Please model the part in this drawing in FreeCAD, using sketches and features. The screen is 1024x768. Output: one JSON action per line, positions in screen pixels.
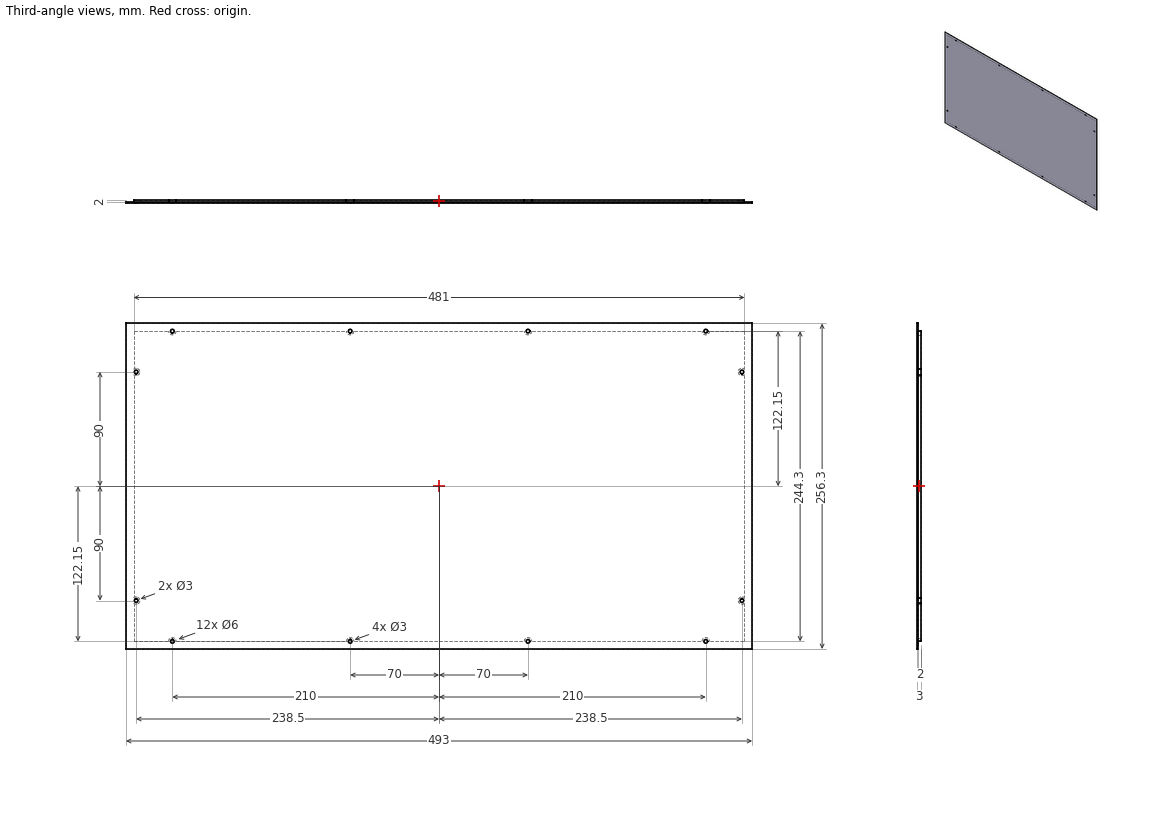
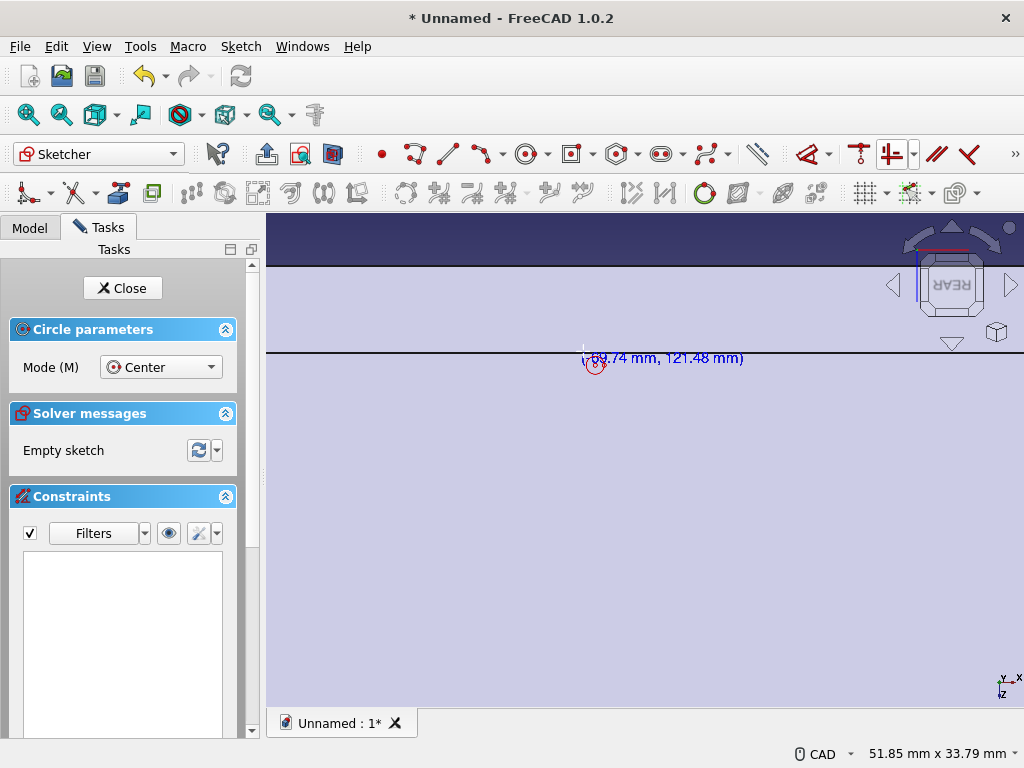
{"action": "scroll", "coordinate": [511, 409], "scroll_direction": "down", "scroll_amount": 15}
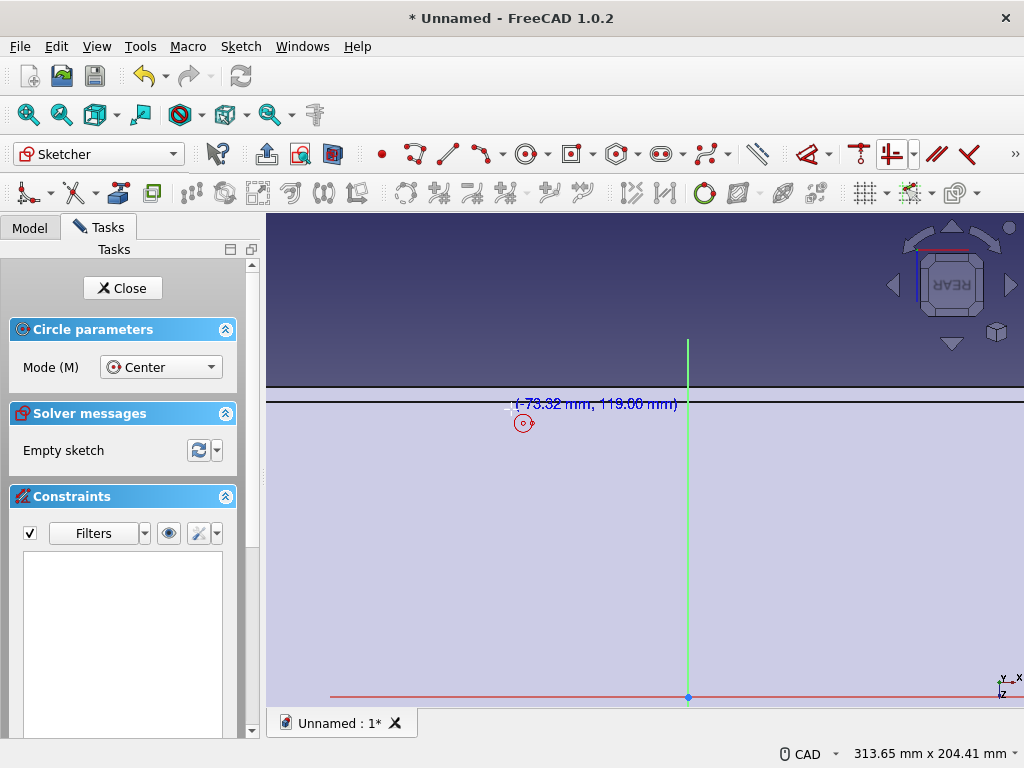
{"action": "left_click", "coordinate": [514, 407]}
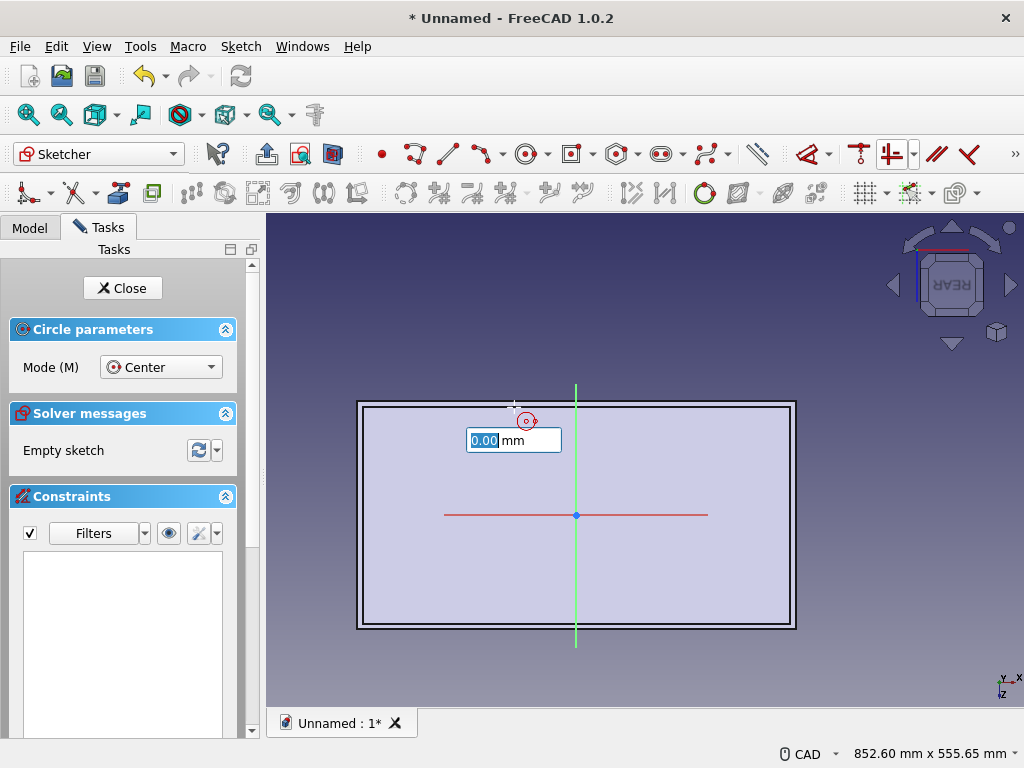
{"action": "scroll", "coordinate": [515, 406], "scroll_direction": "up", "scroll_amount": 13}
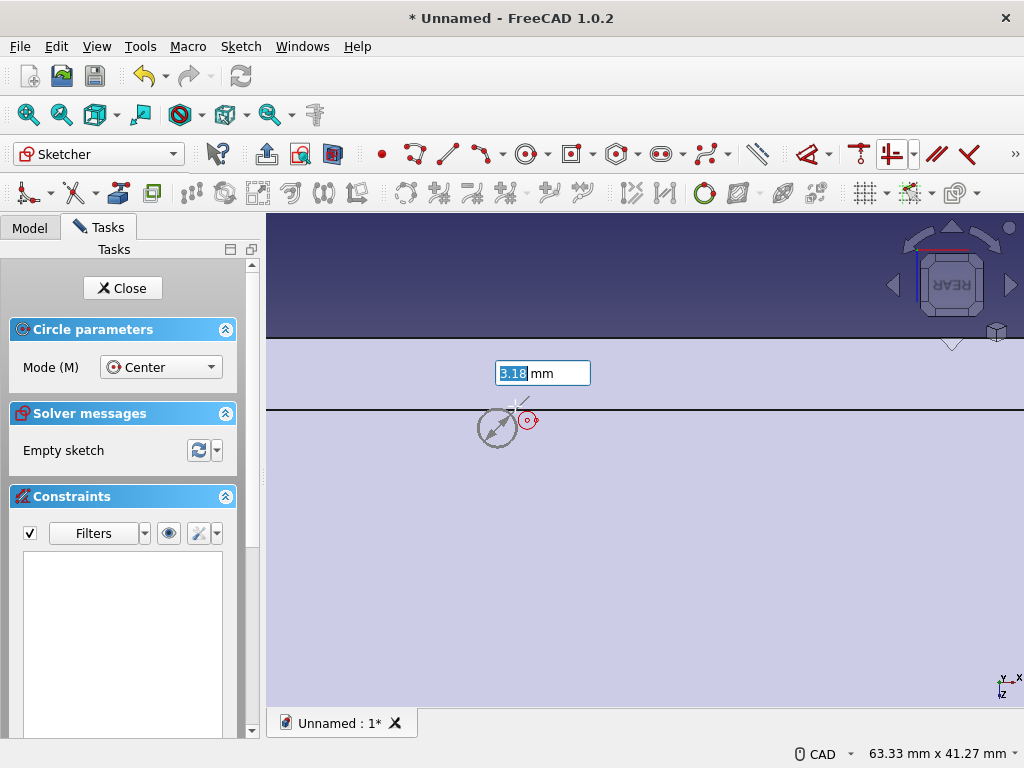
{"action": "left_click", "coordinate": [514, 397]}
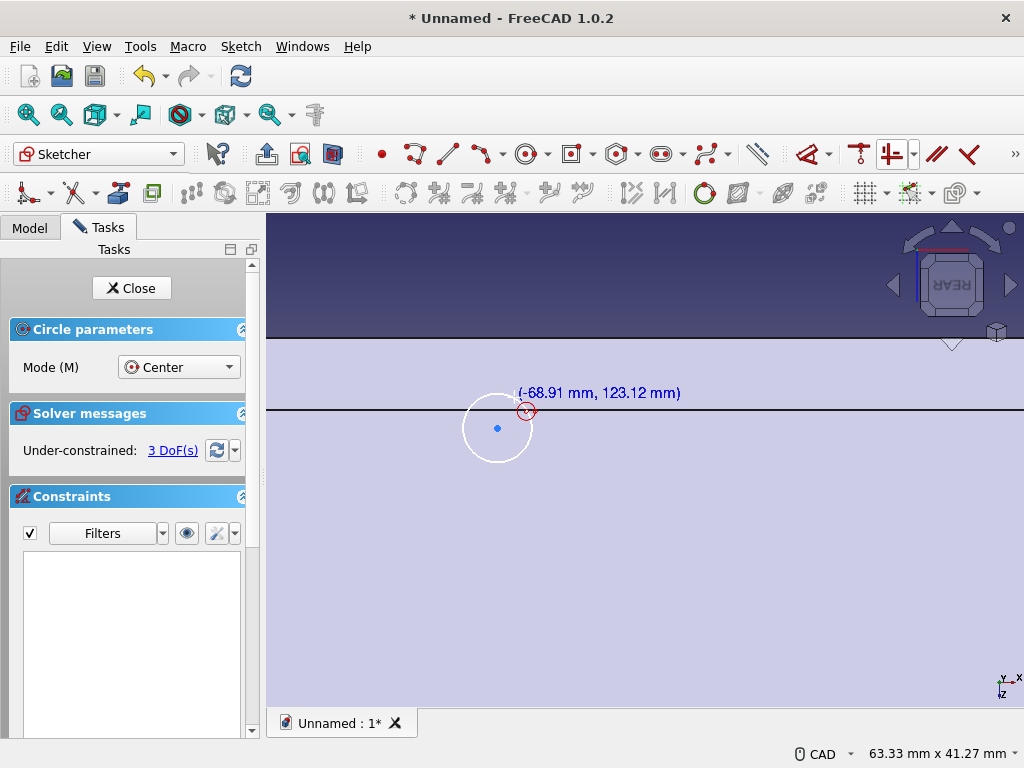
{"action": "scroll", "coordinate": [515, 406], "scroll_direction": "down", "scroll_amount": 13}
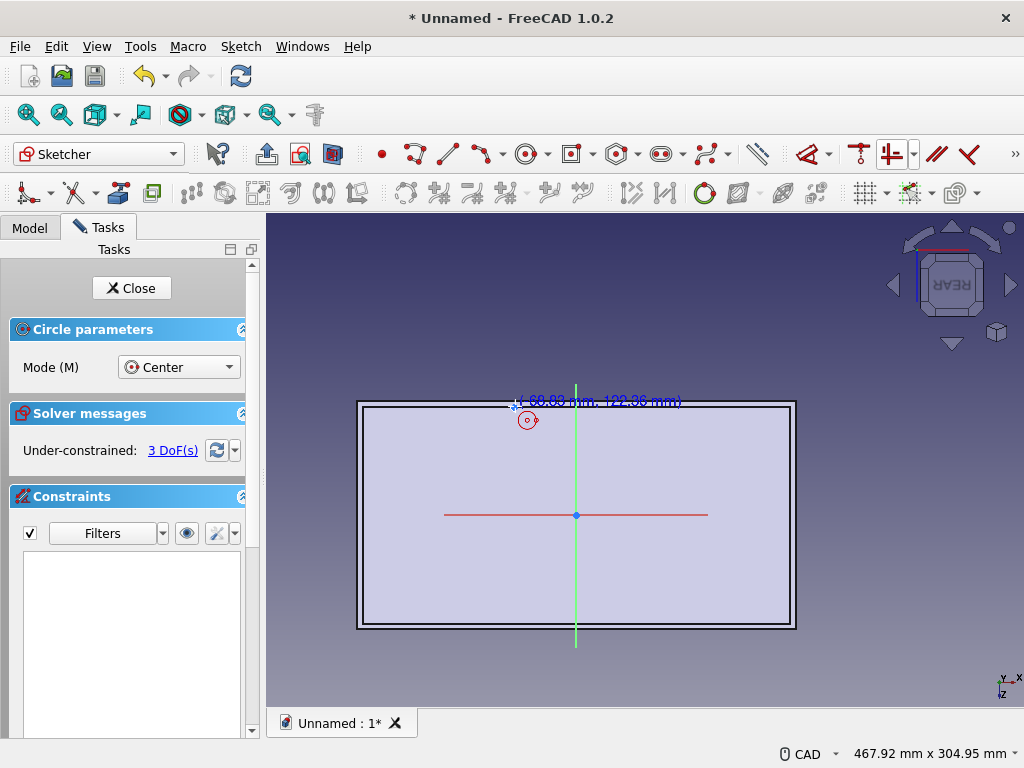
{"action": "scroll", "coordinate": [390, 407], "scroll_direction": "up", "scroll_amount": 15}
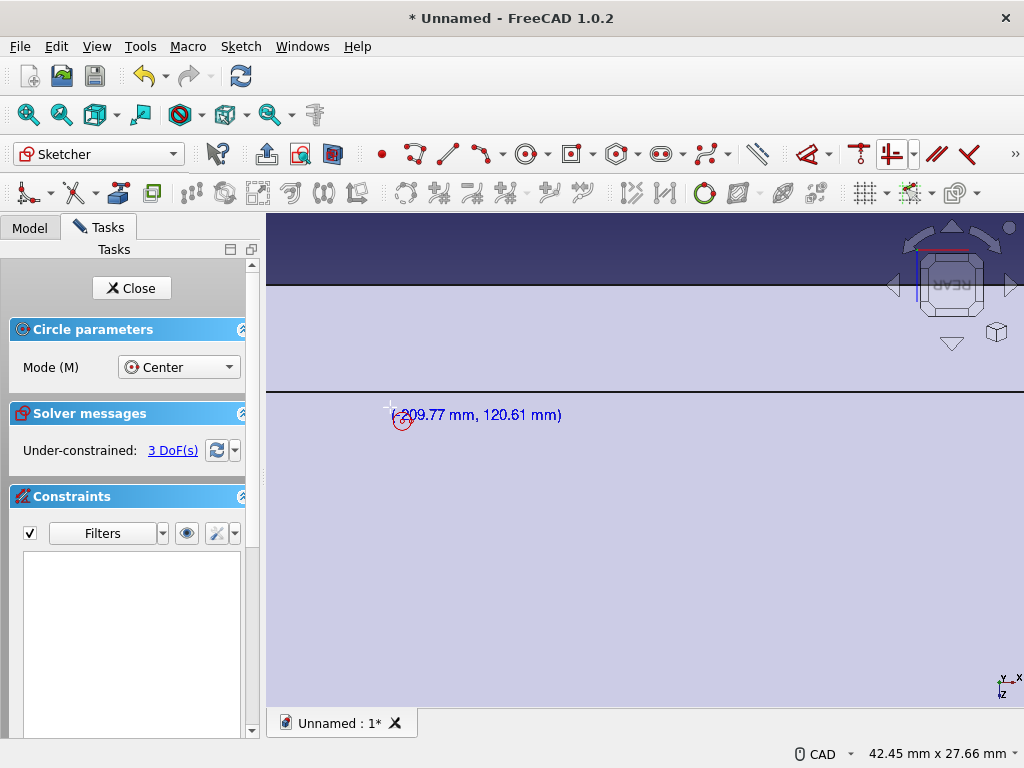
{"action": "scroll", "coordinate": [390, 407], "scroll_direction": "down", "scroll_amount": 15}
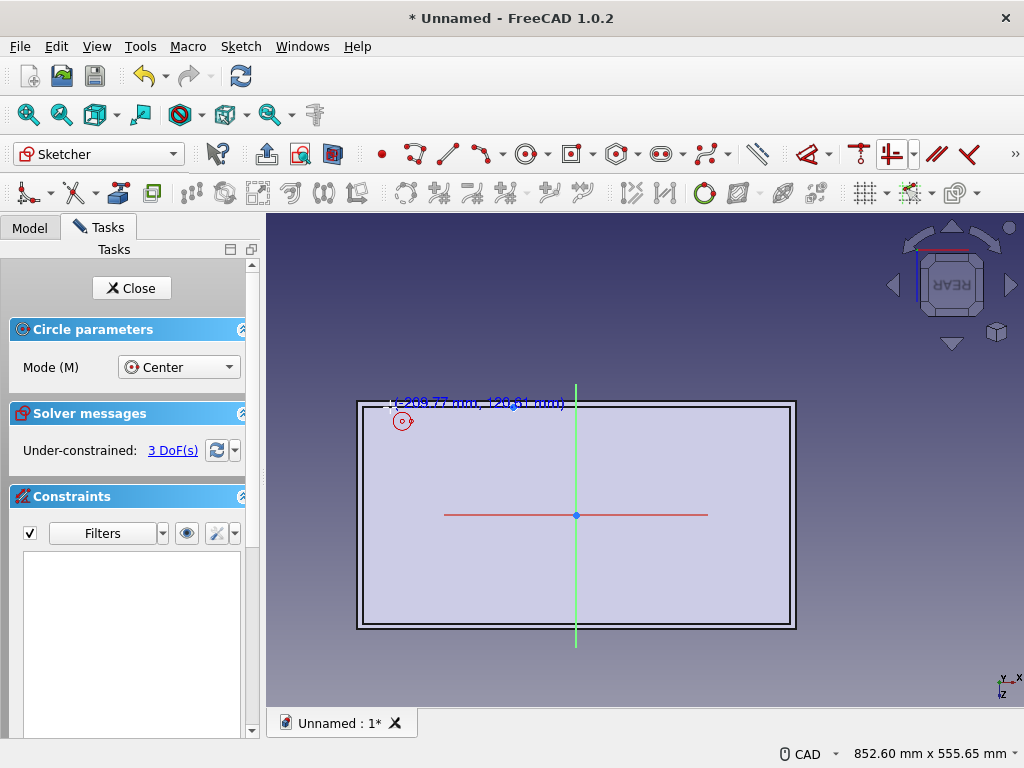
{"action": "left_click", "coordinate": [390, 407]}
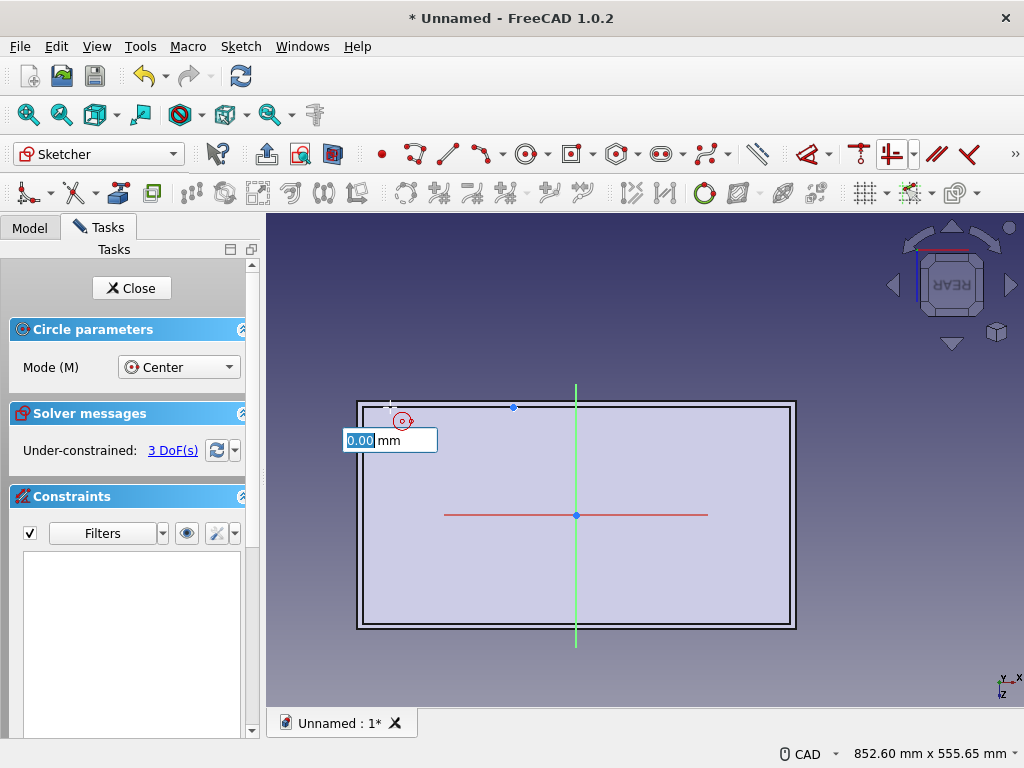
{"action": "scroll", "coordinate": [391, 406], "scroll_direction": "up", "scroll_amount": 13}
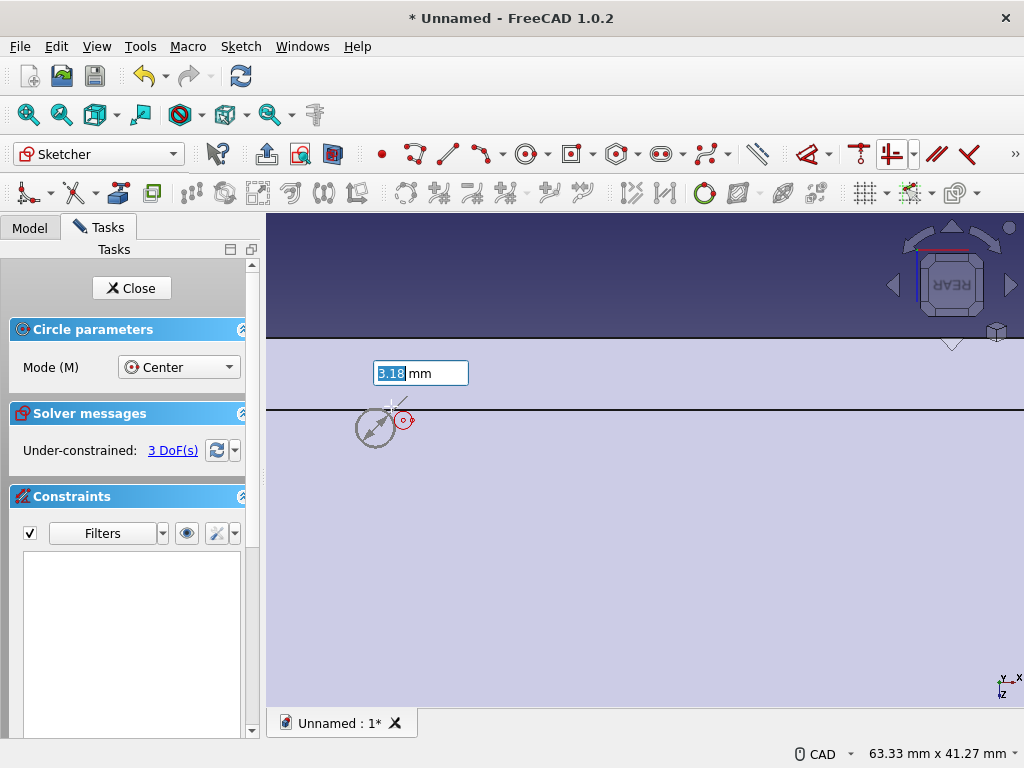
{"action": "left_click", "coordinate": [385, 397]}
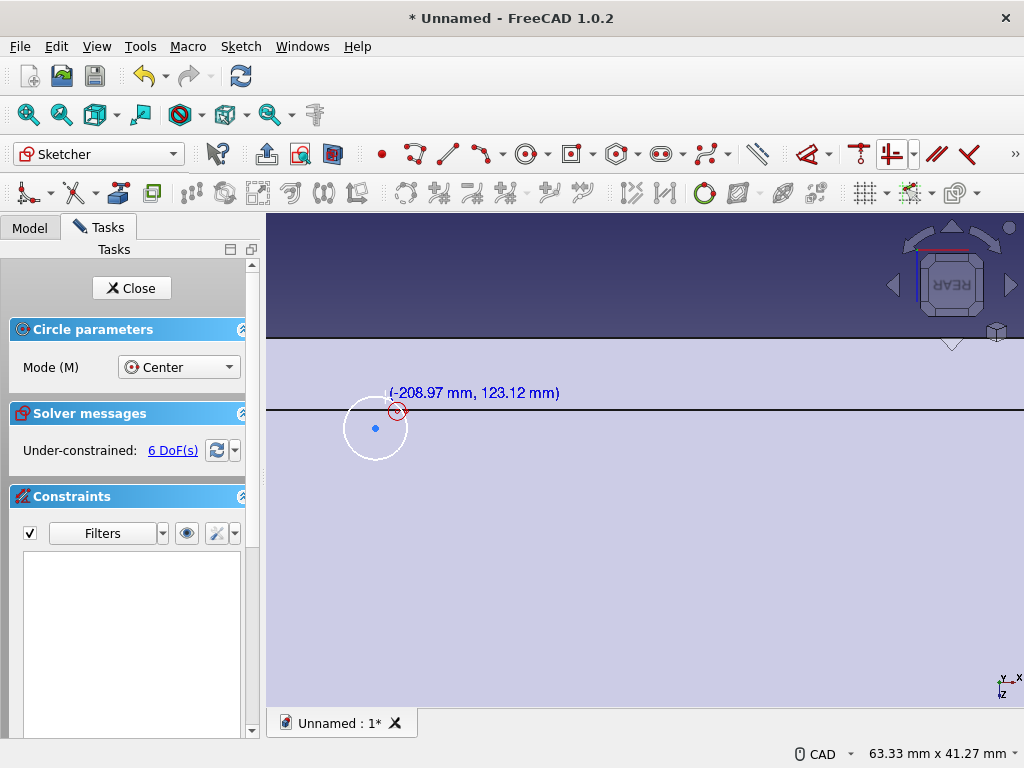
{"action": "scroll", "coordinate": [391, 406], "scroll_direction": "down", "scroll_amount": 13}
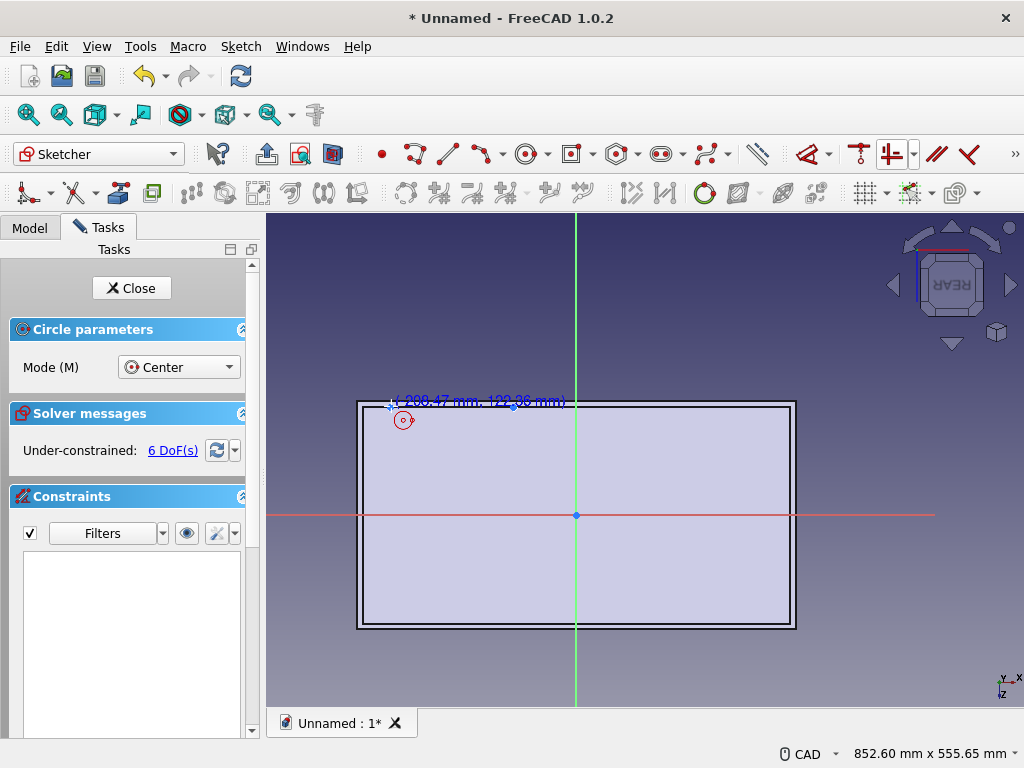
{"action": "scroll", "coordinate": [639, 407], "scroll_direction": "up", "scroll_amount": 15}